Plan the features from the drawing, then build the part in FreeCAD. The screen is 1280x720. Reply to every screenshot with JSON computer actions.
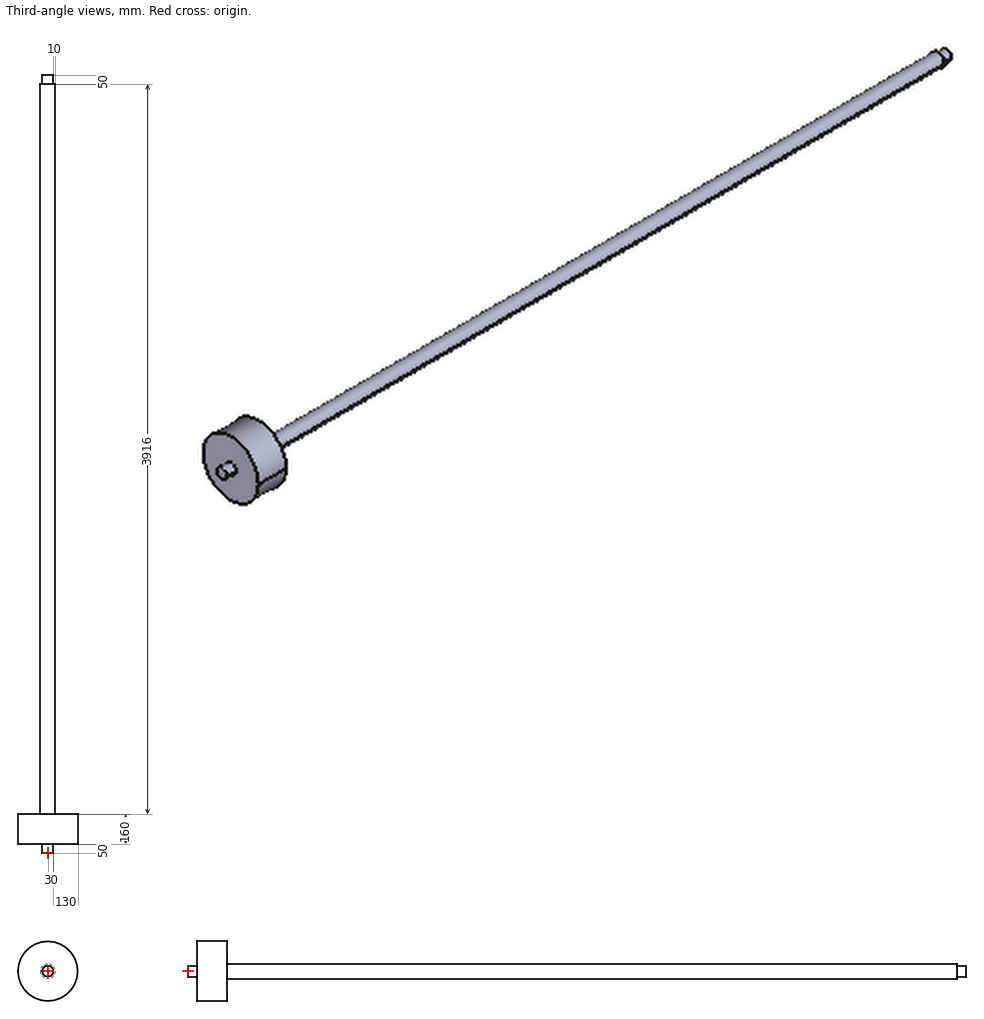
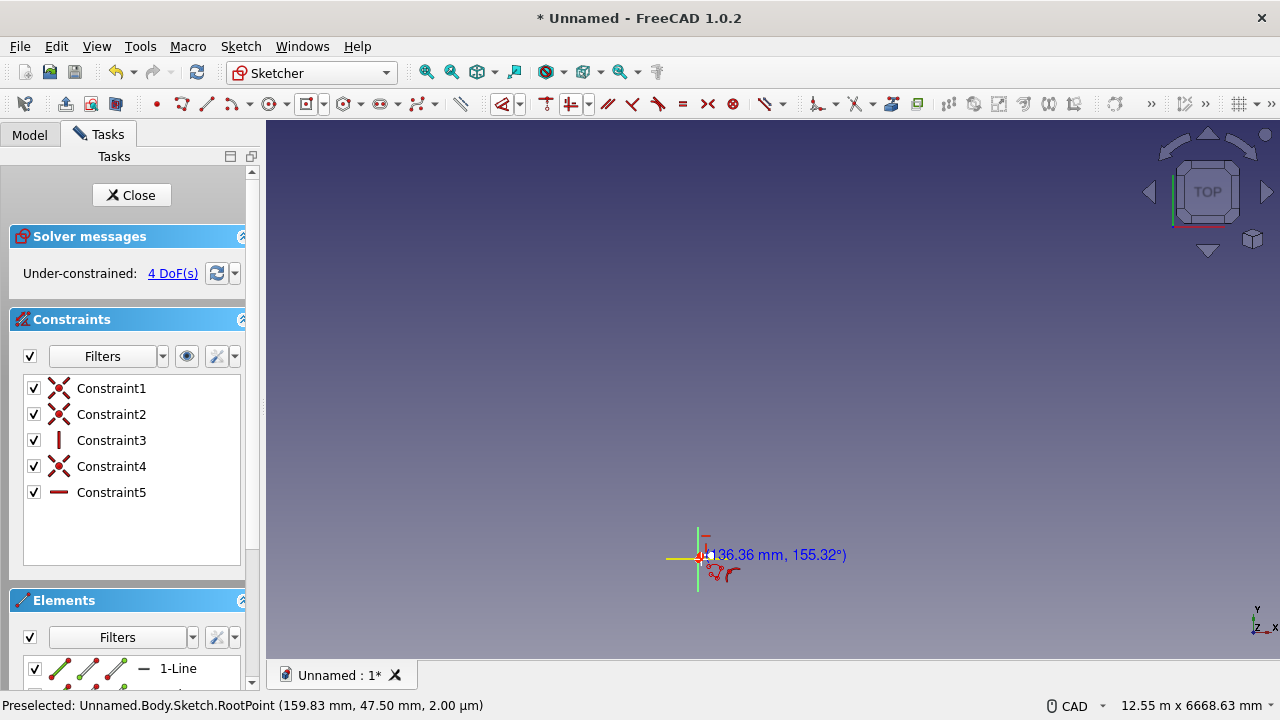
{"action": "scroll", "coordinate": [711, 542], "scroll_direction": "up", "scroll_amount": 2}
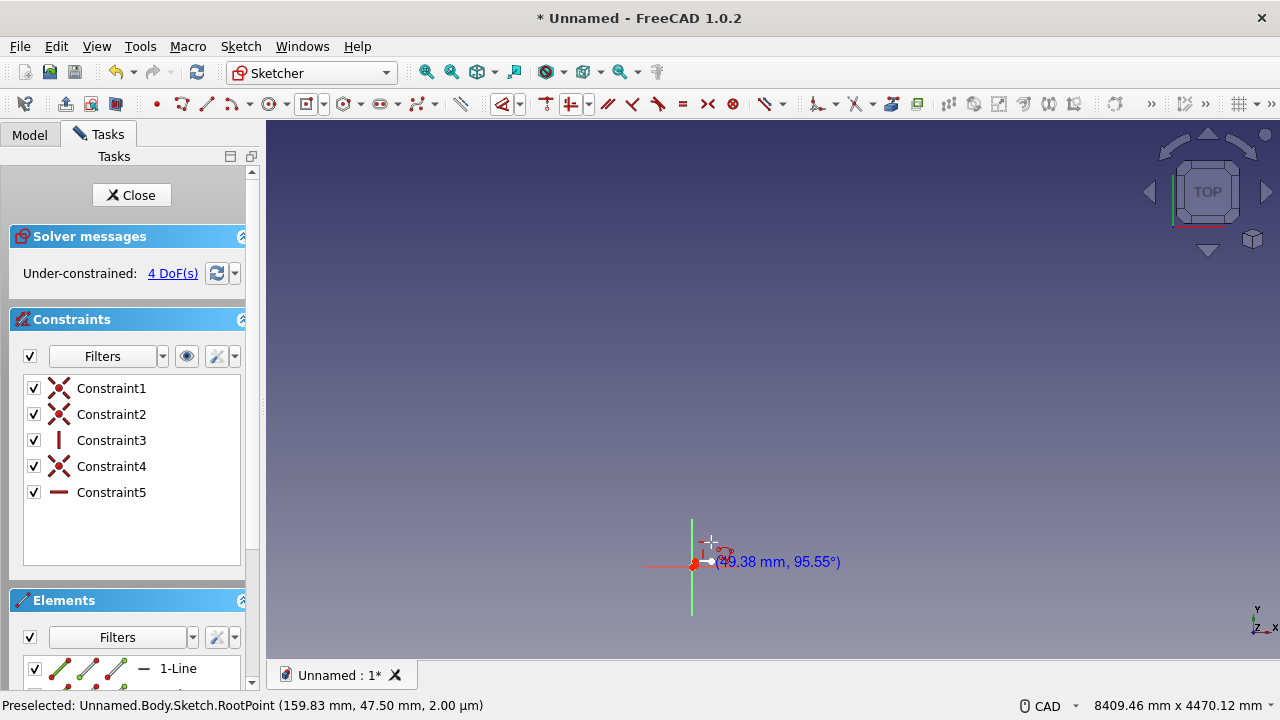
{"action": "left_click", "coordinate": [711, 542]}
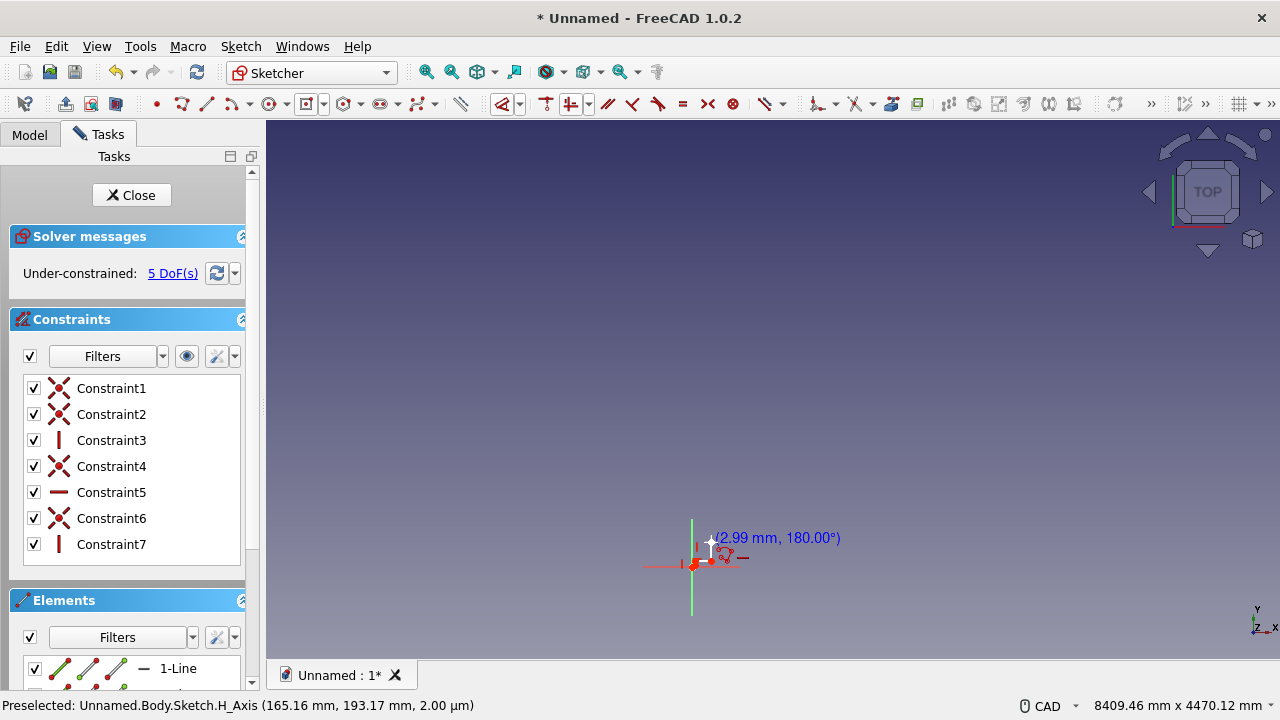
{"action": "scroll", "coordinate": [697, 542], "scroll_direction": "up", "scroll_amount": 6}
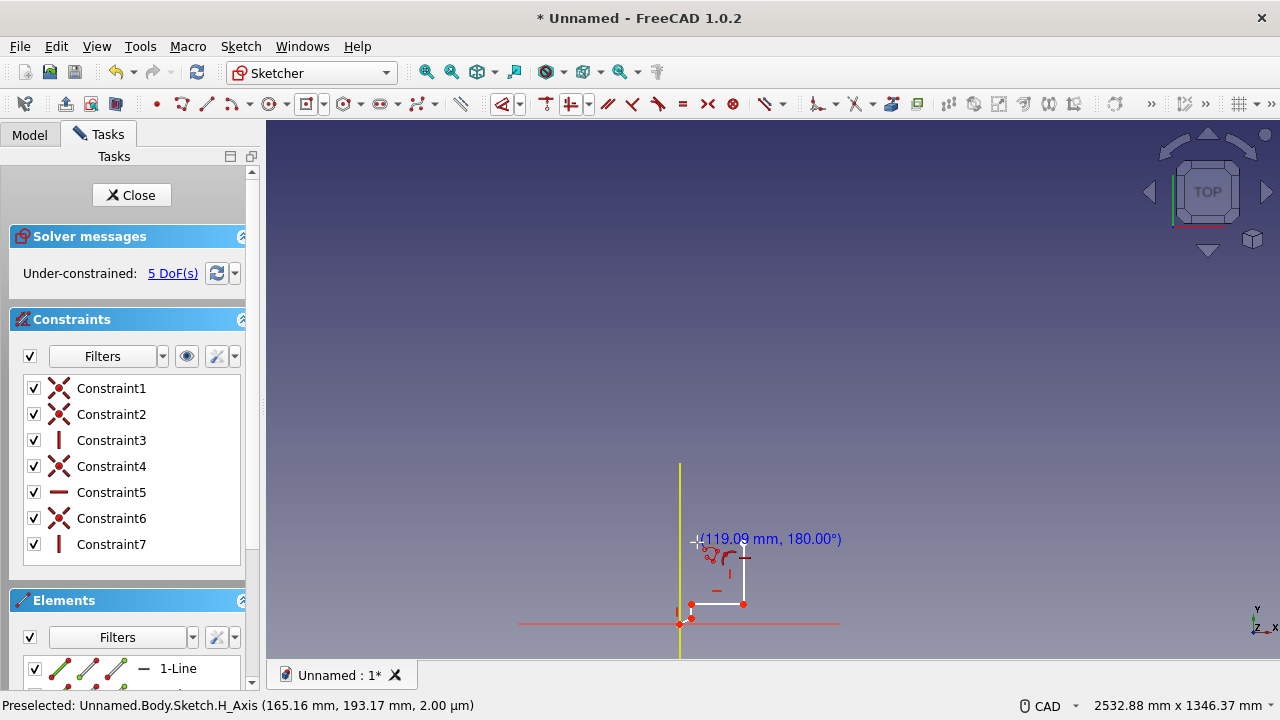
{"action": "left_click", "coordinate": [696, 540]}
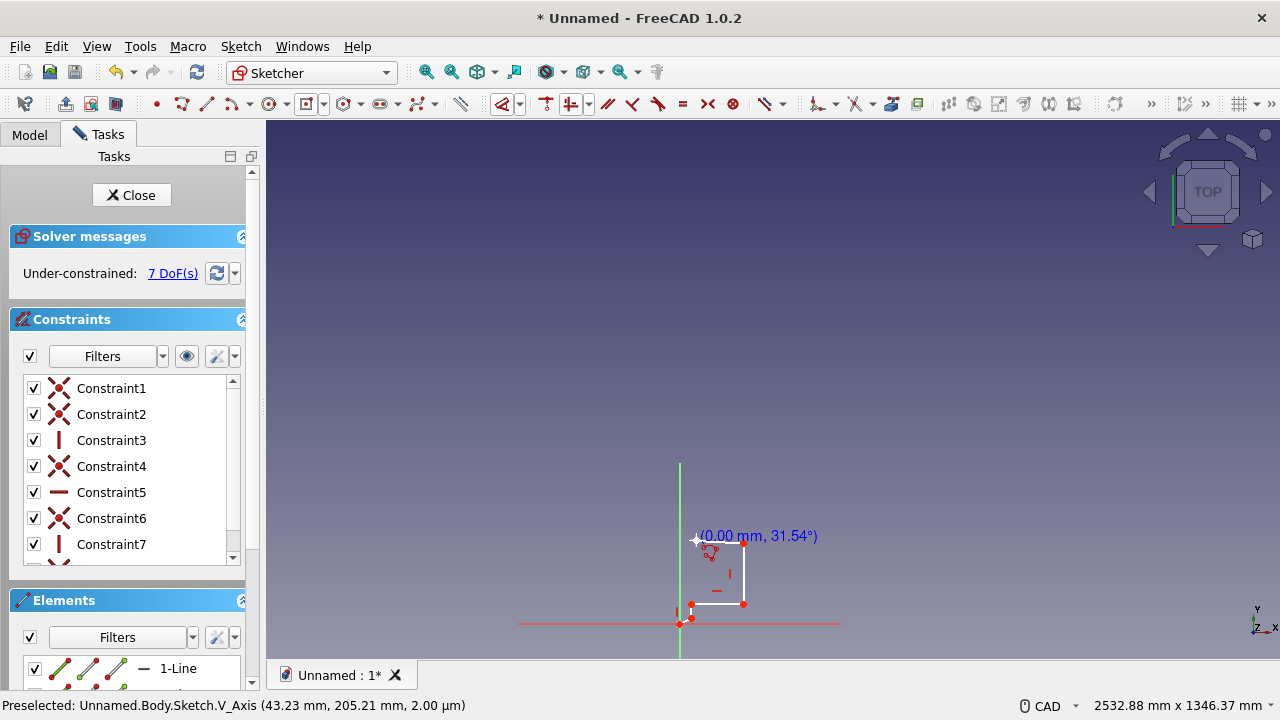
{"action": "scroll", "coordinate": [703, 542], "scroll_direction": "down", "scroll_amount": 8}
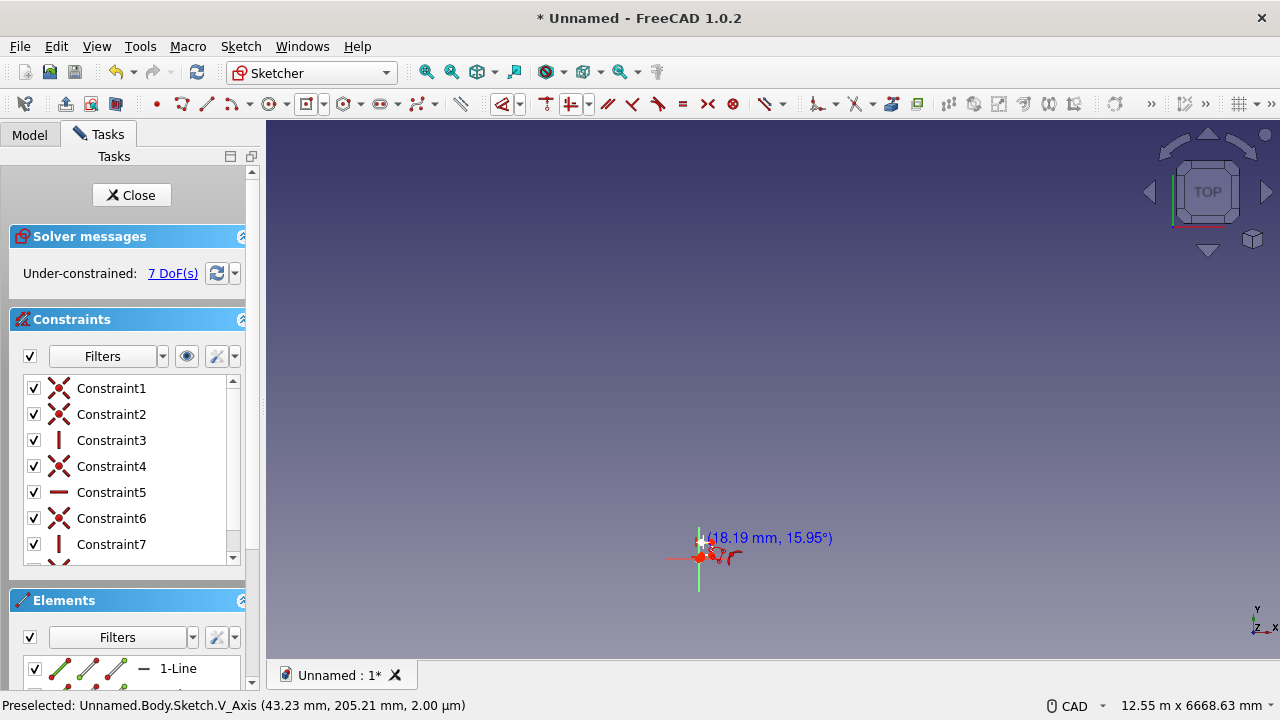
{"action": "scroll", "coordinate": [702, 226], "scroll_direction": "up", "scroll_amount": 8}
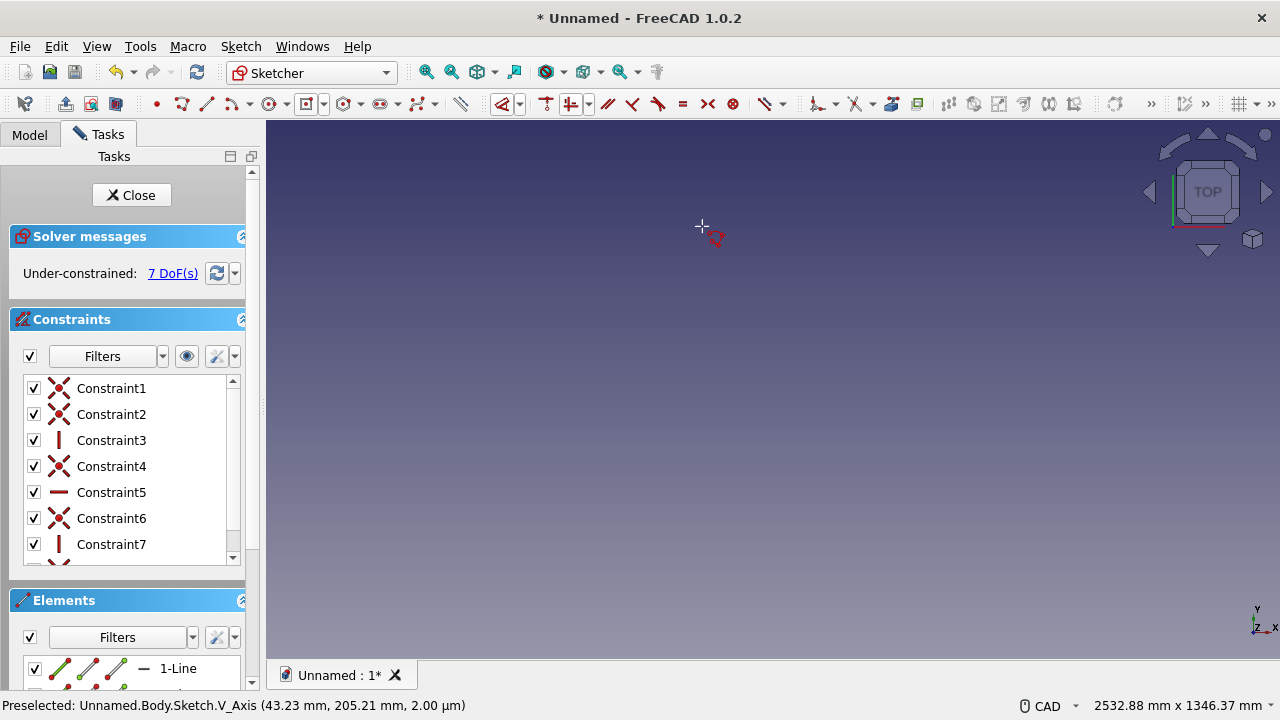
{"action": "left_click", "coordinate": [700, 224]}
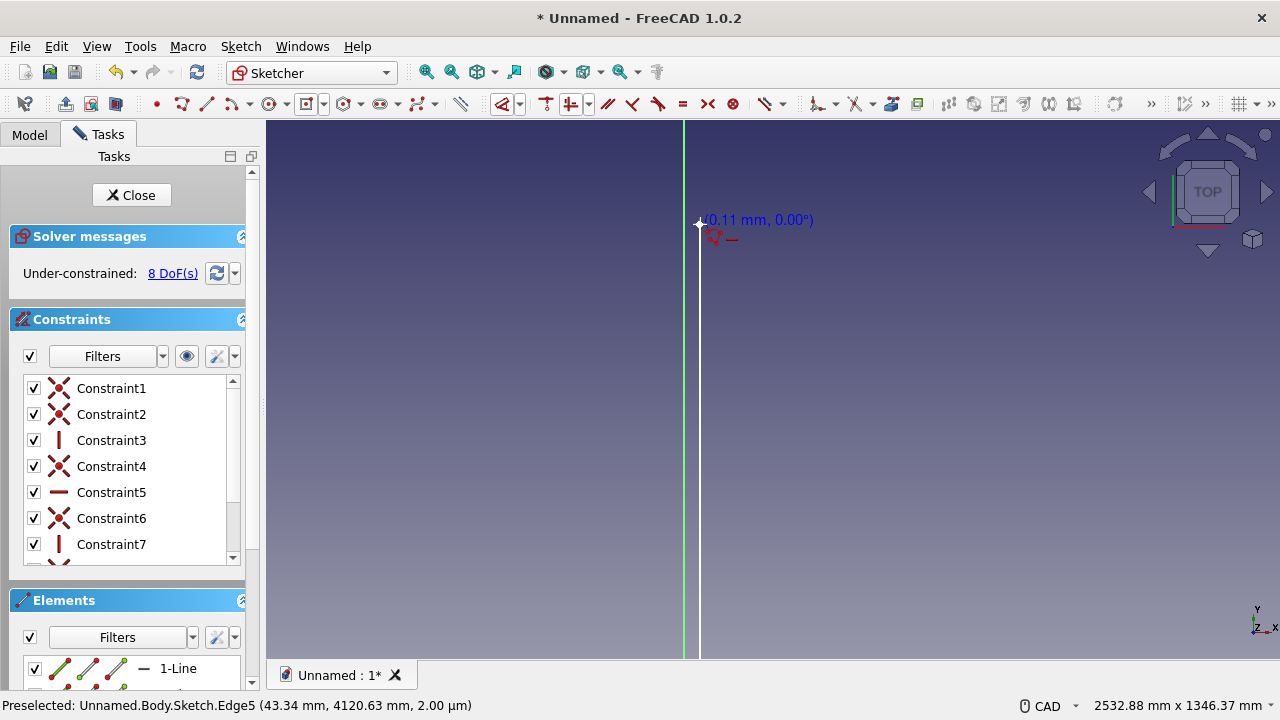
{"action": "scroll", "coordinate": [696, 224], "scroll_direction": "up", "scroll_amount": 7}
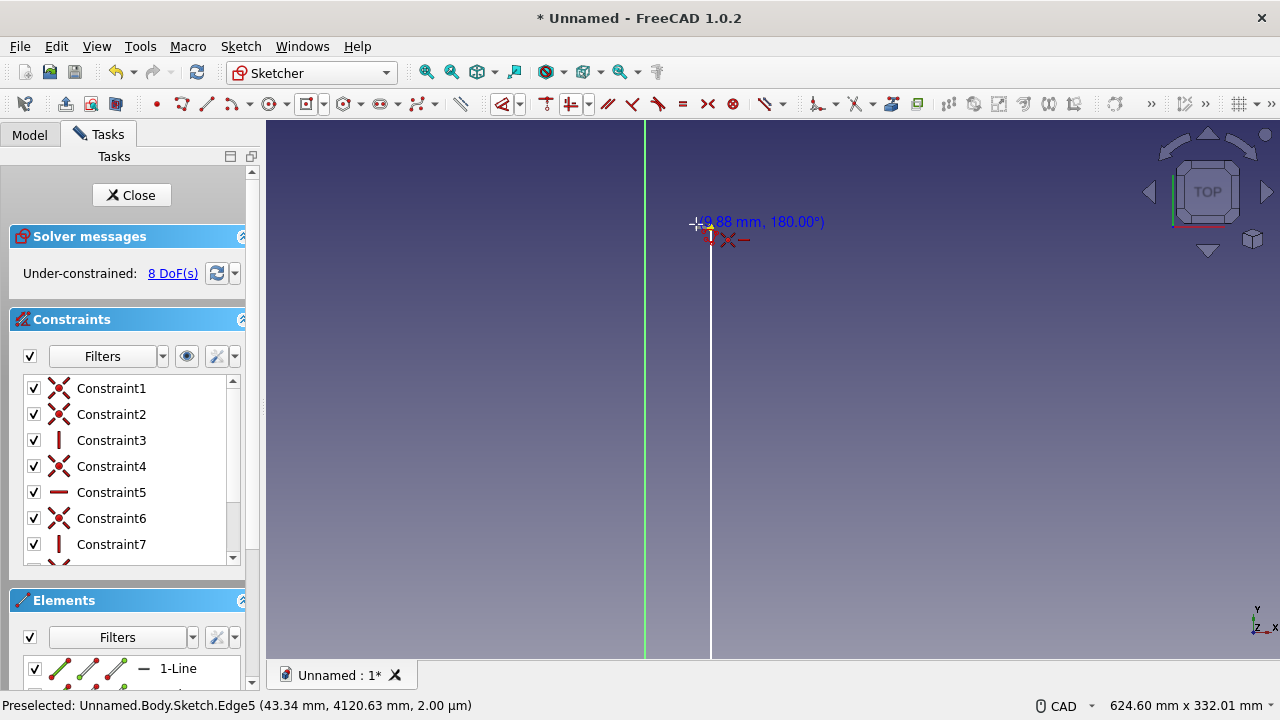
{"action": "left_click", "coordinate": [693, 223]}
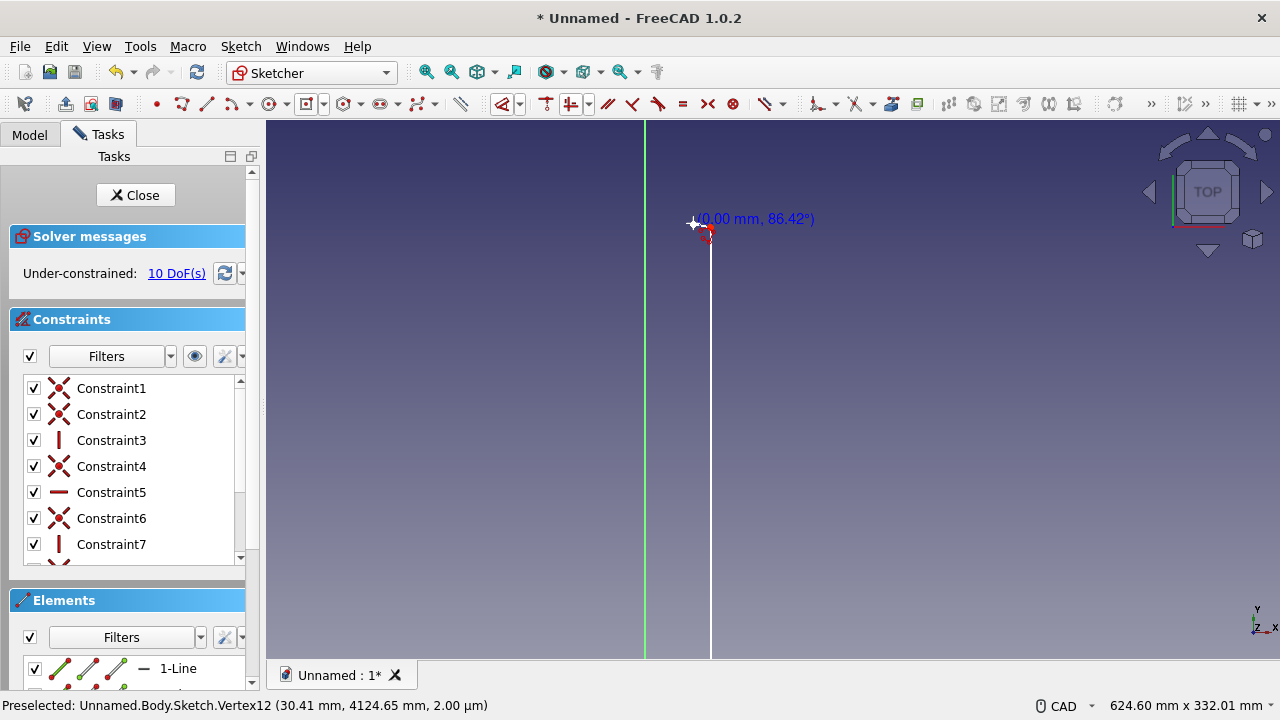
{"action": "scroll", "coordinate": [701, 225], "scroll_direction": "down", "scroll_amount": 15}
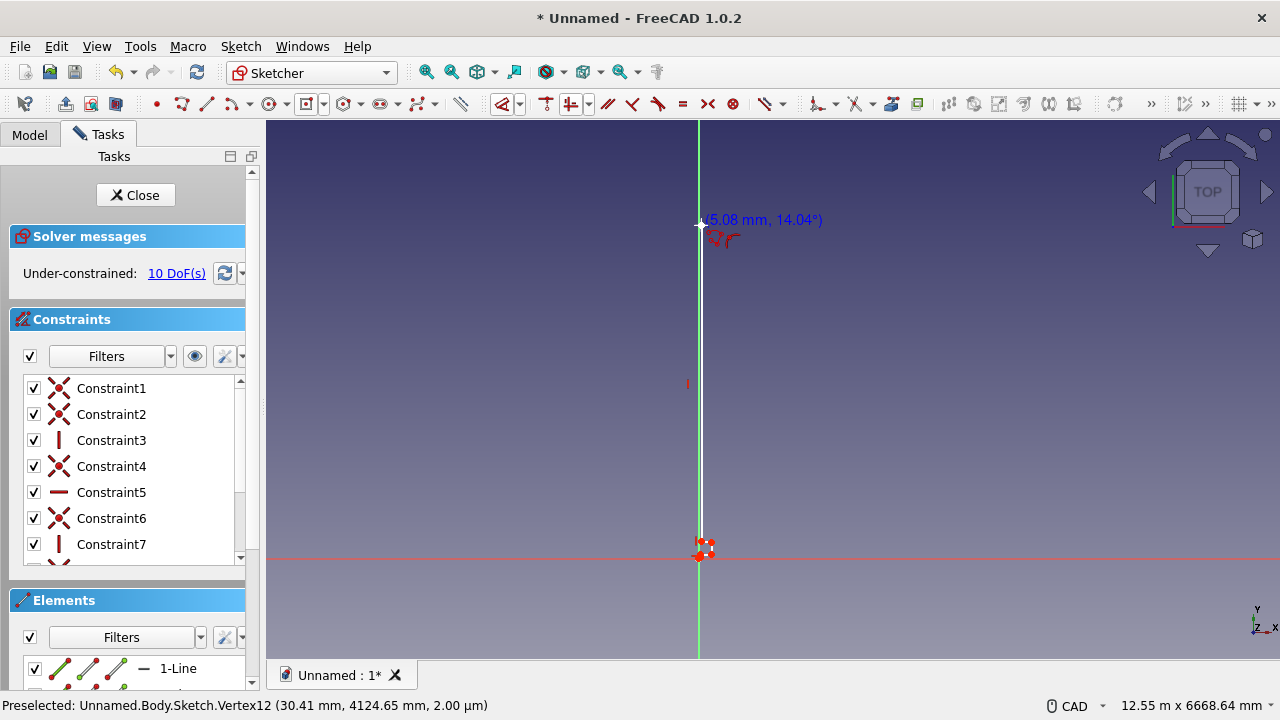
{"action": "scroll", "coordinate": [701, 221], "scroll_direction": "up", "scroll_amount": 10}